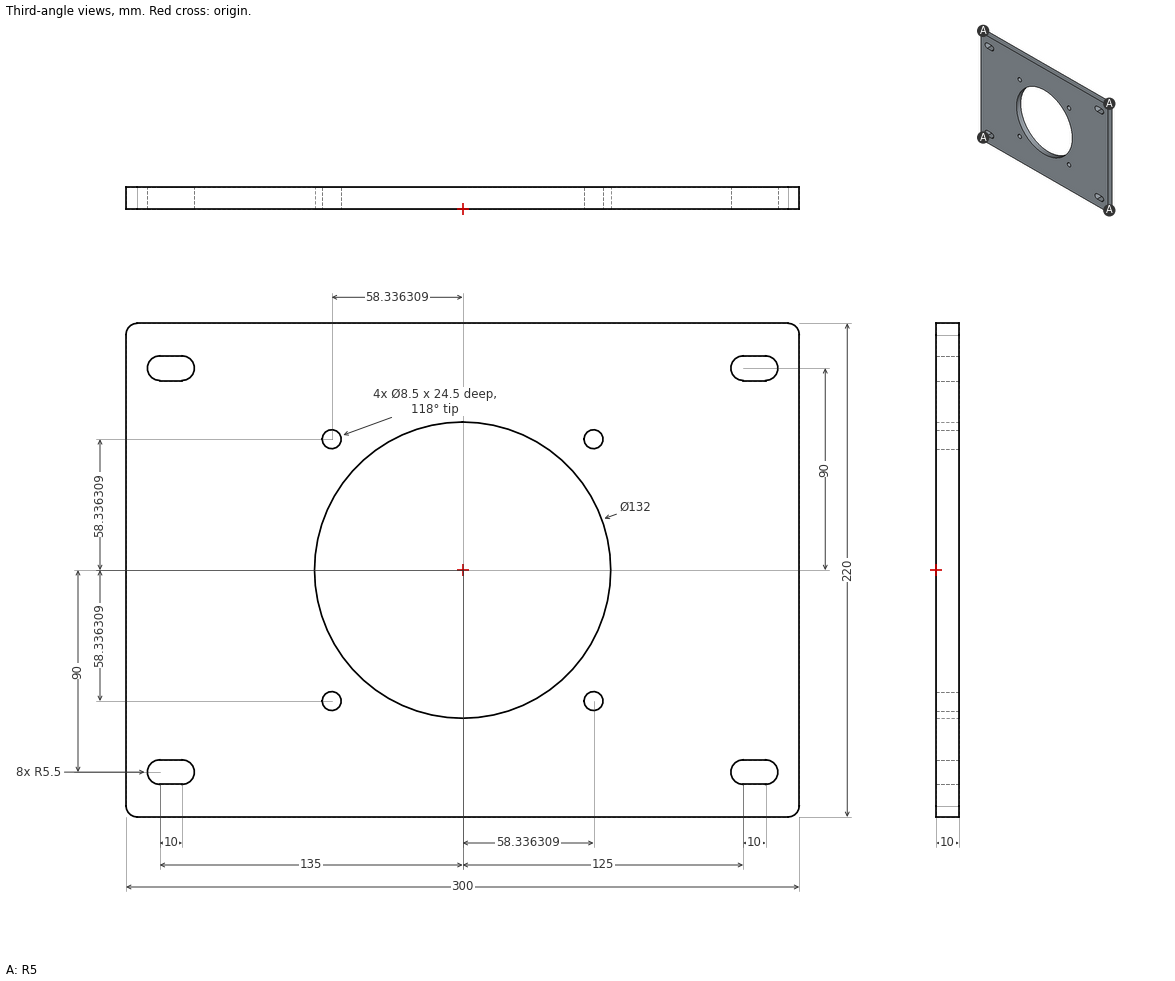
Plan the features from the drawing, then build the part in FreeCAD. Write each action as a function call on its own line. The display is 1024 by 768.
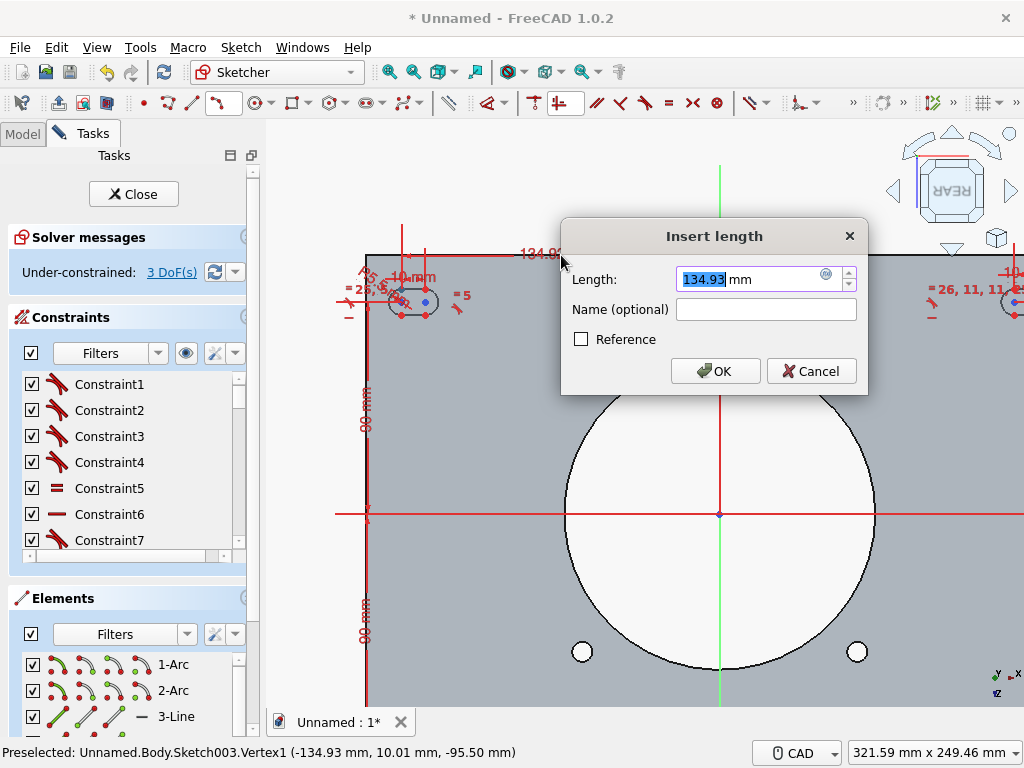
text(135)
key(Return)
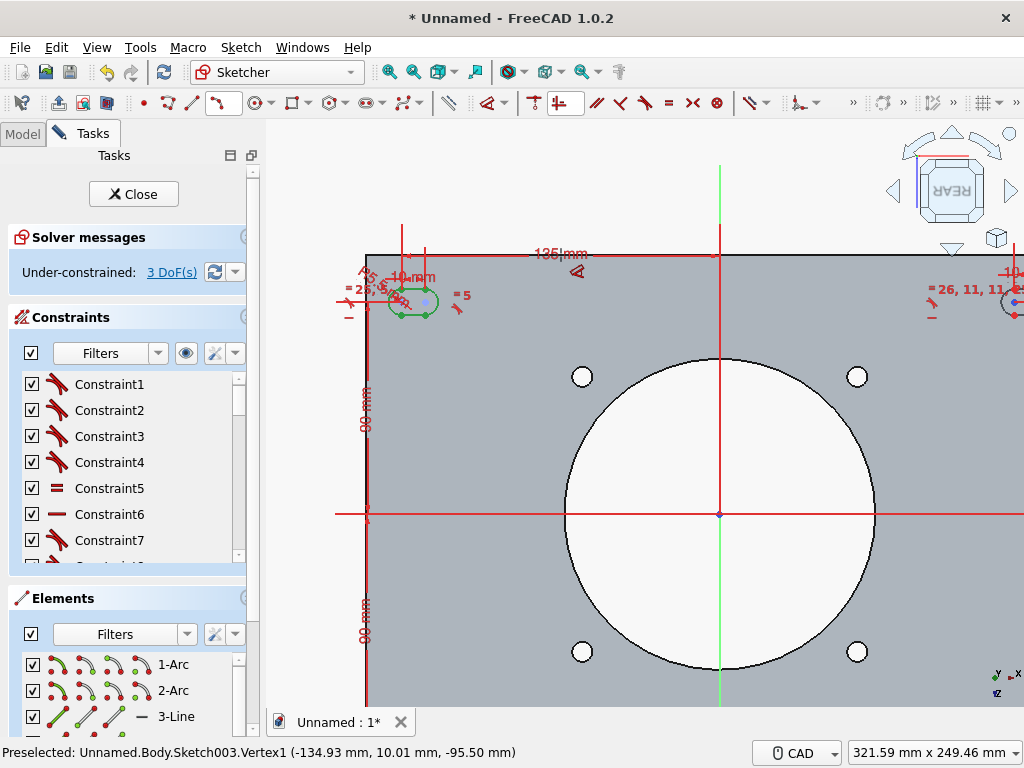
scroll(402, 290, down, 3)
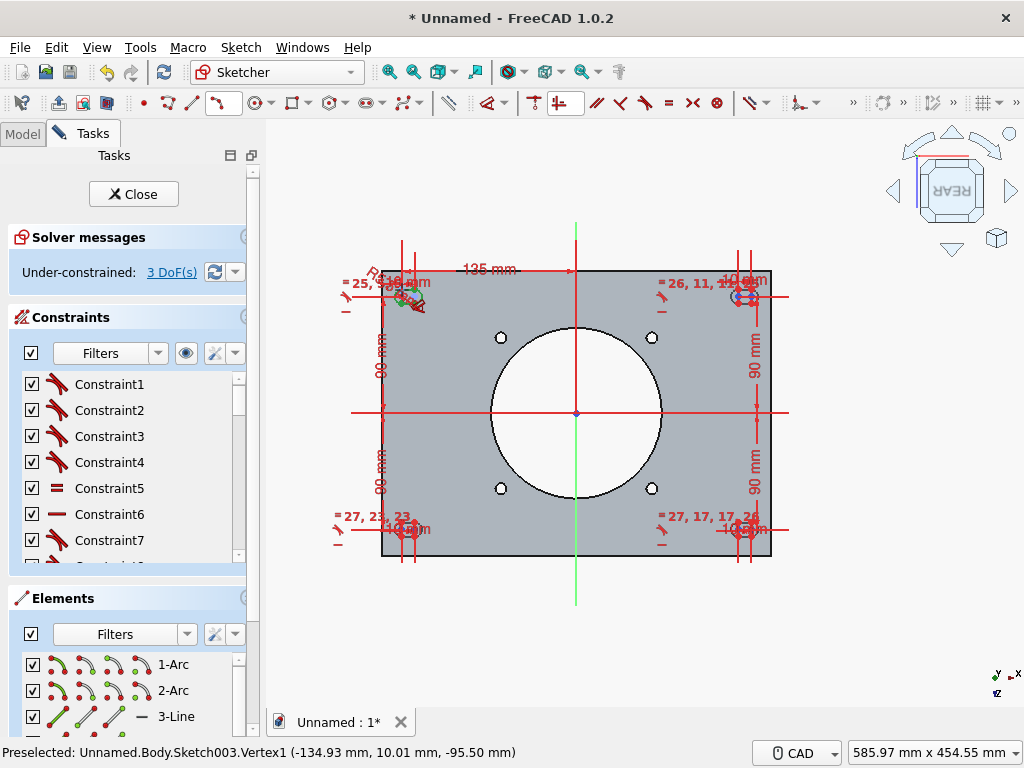
scroll(738, 290, up, 3)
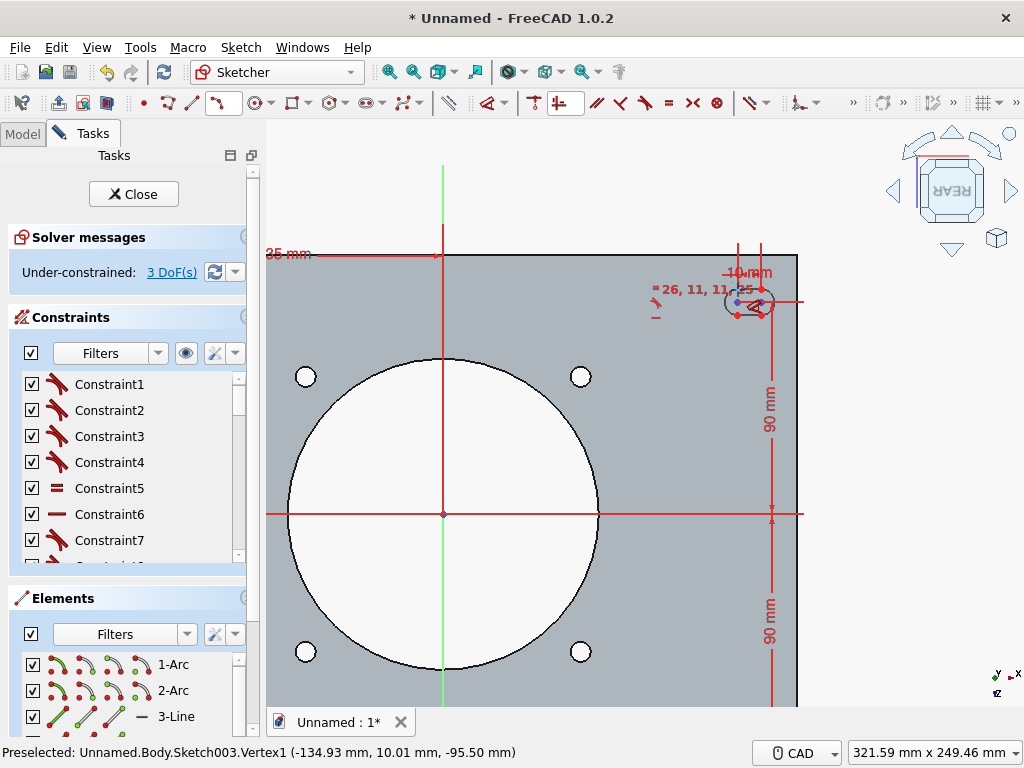
click(738, 289)
click(590, 255)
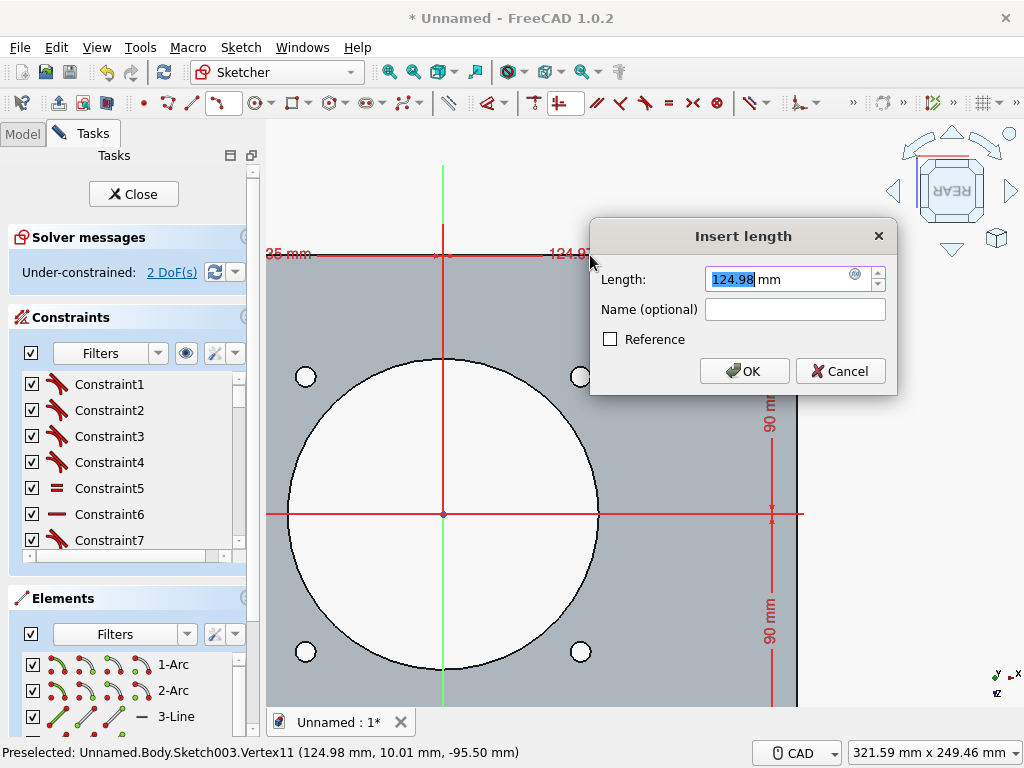
text(125)
key(Return)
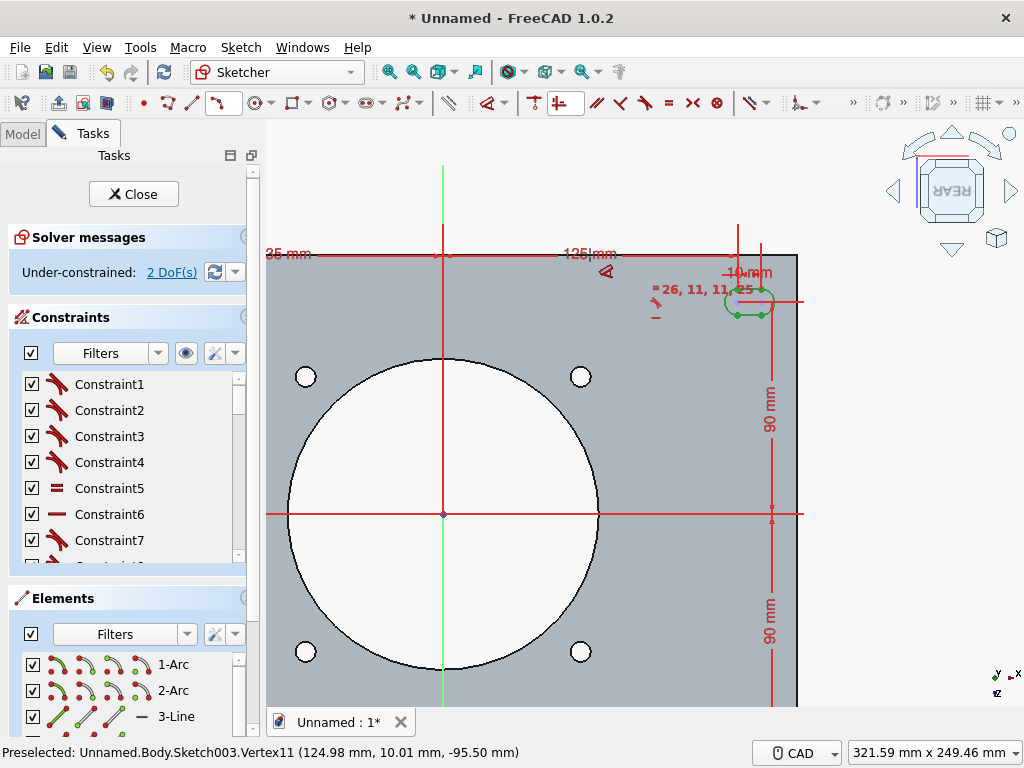
scroll(739, 290, down, 3)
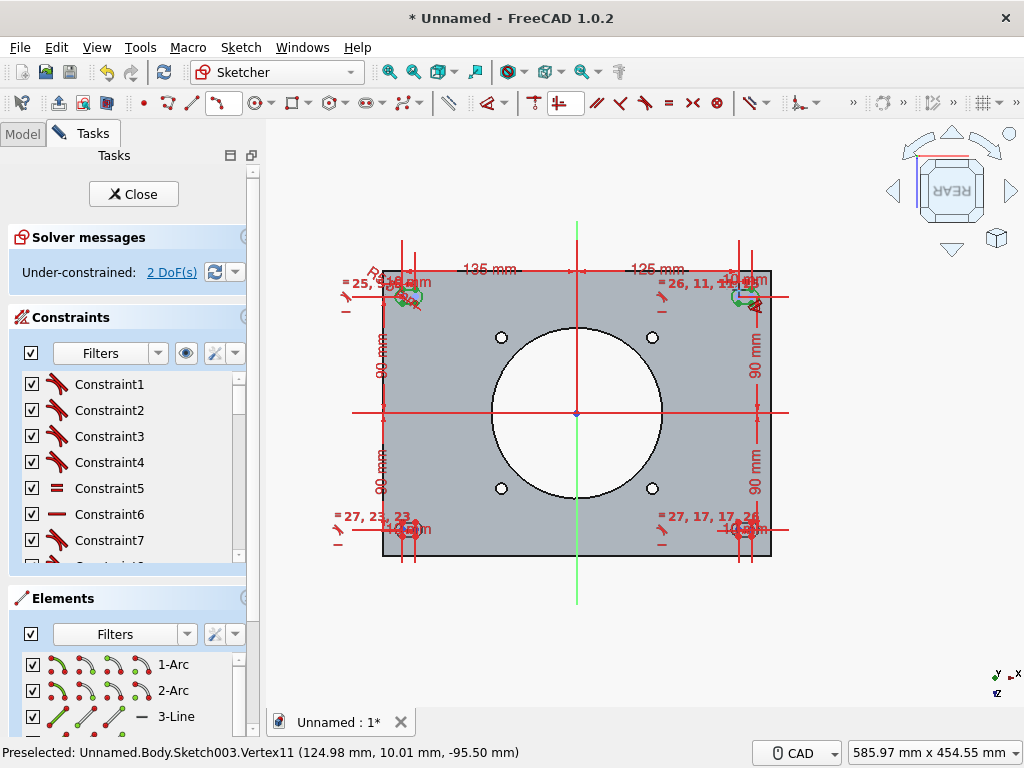
scroll(739, 523, up, 3)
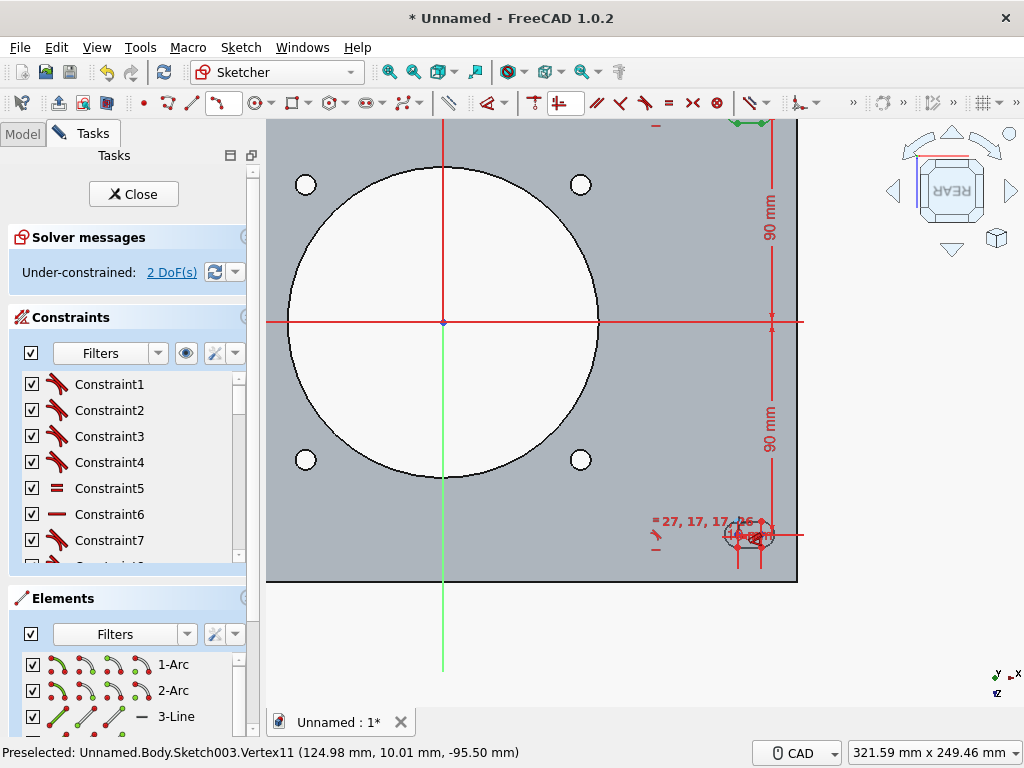
click(738, 522)
click(590, 556)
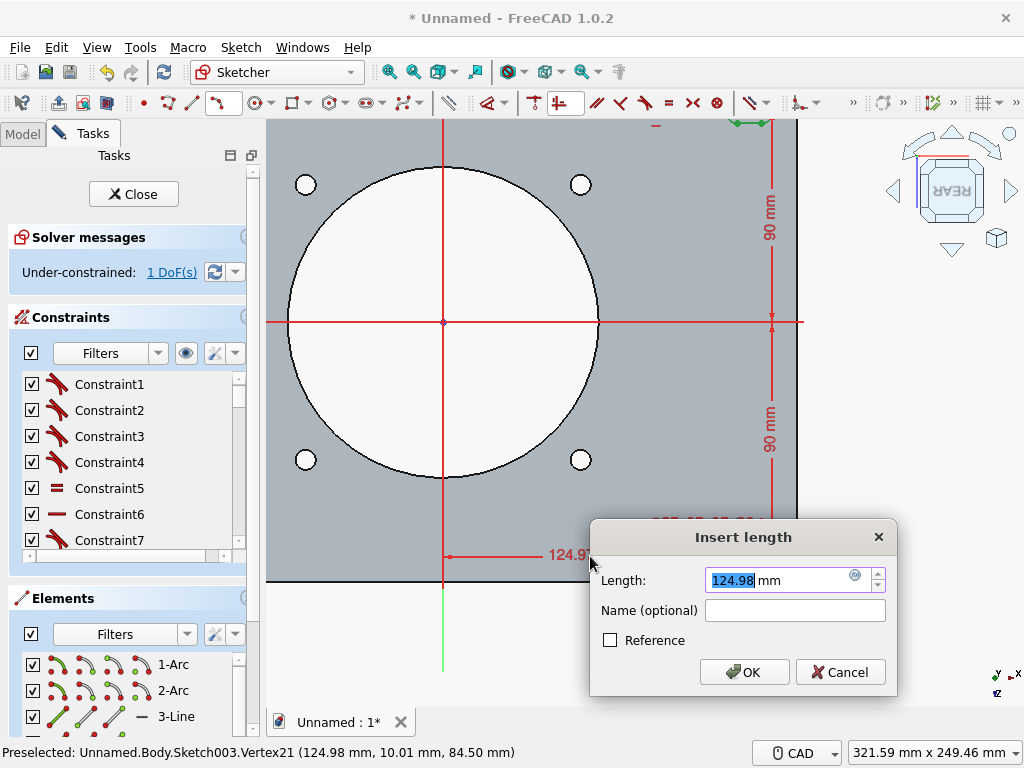
text(125)
key(Return)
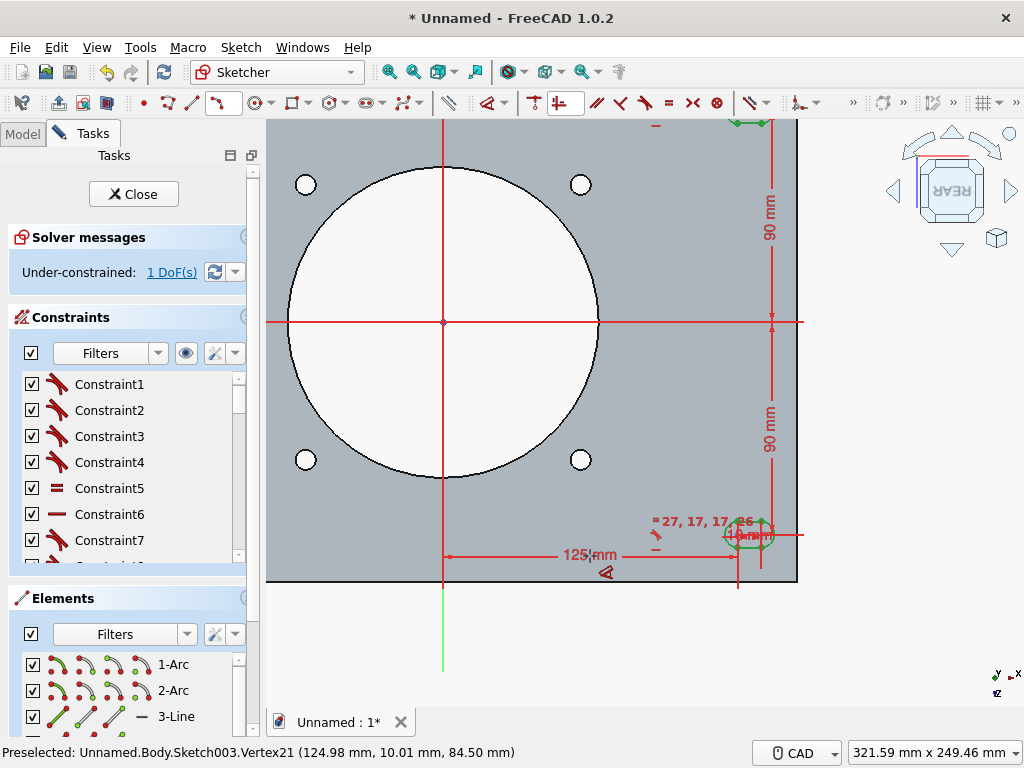
scroll(739, 523, down, 3)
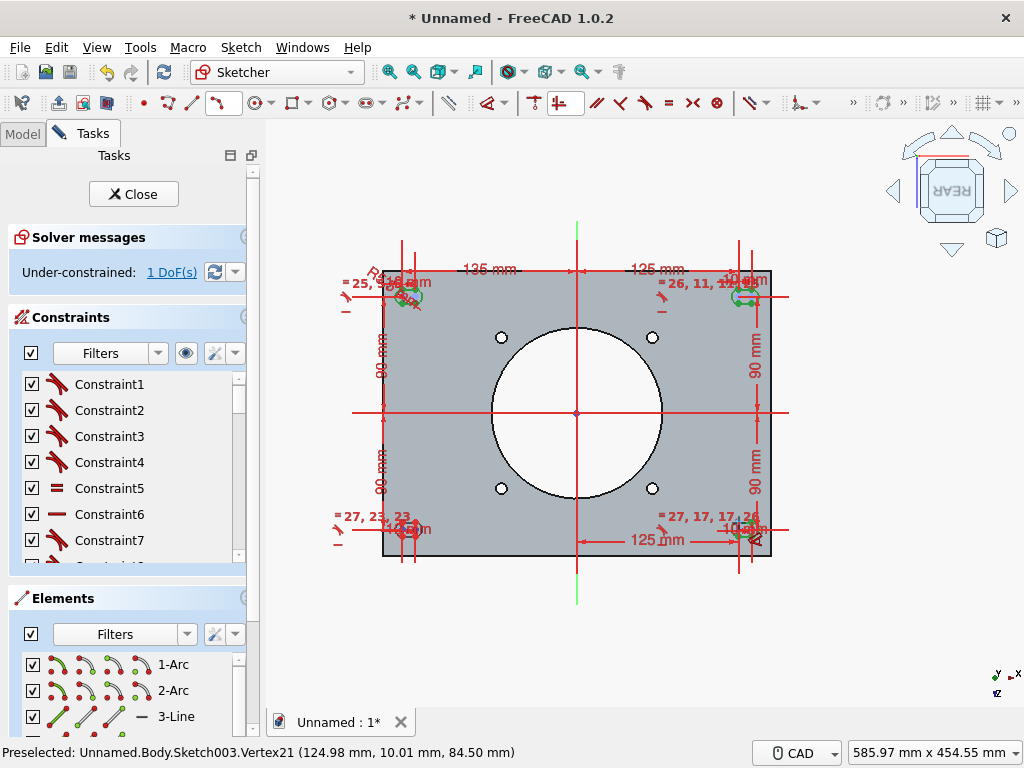
scroll(402, 523, up, 3)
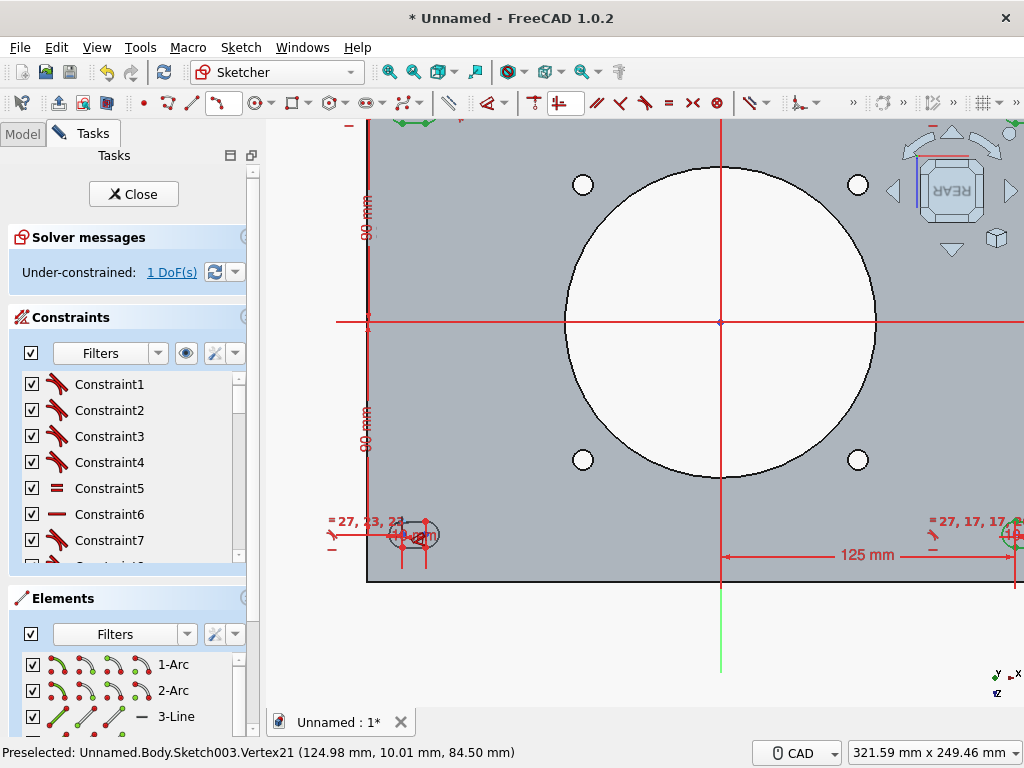
click(402, 522)
click(561, 556)